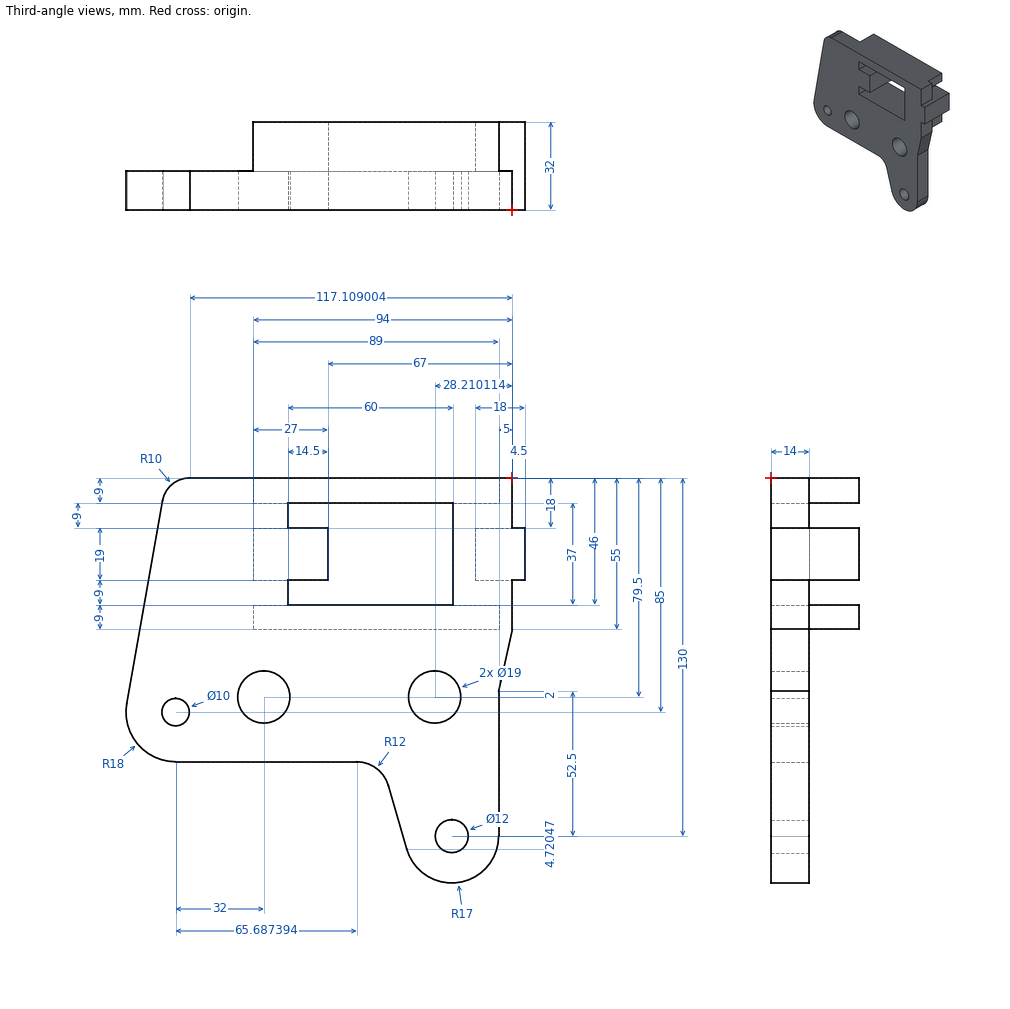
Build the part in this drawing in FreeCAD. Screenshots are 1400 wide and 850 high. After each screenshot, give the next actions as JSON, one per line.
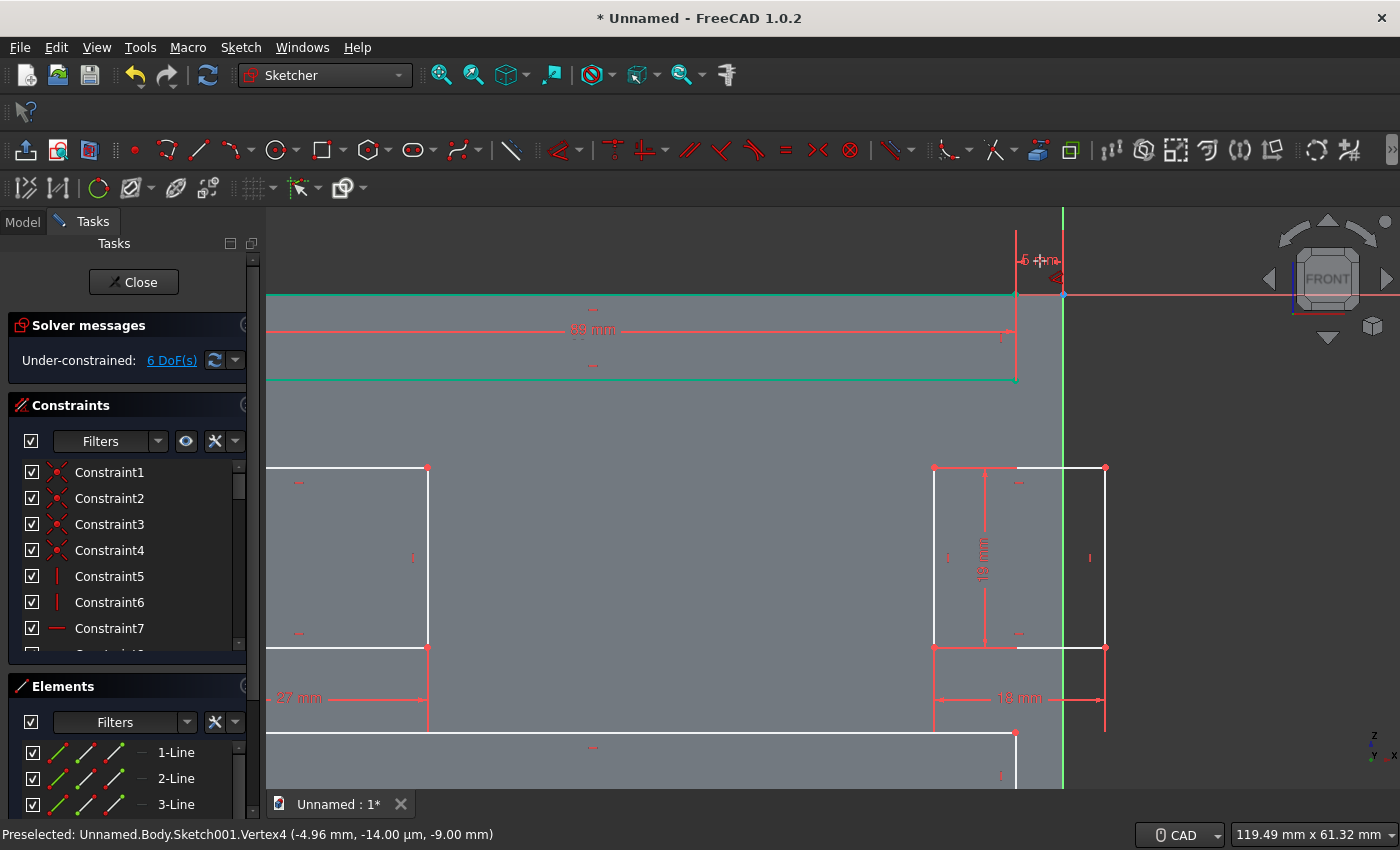
{"action": "scroll", "coordinate": [1021, 381], "scroll_direction": "down", "scroll_amount": 2}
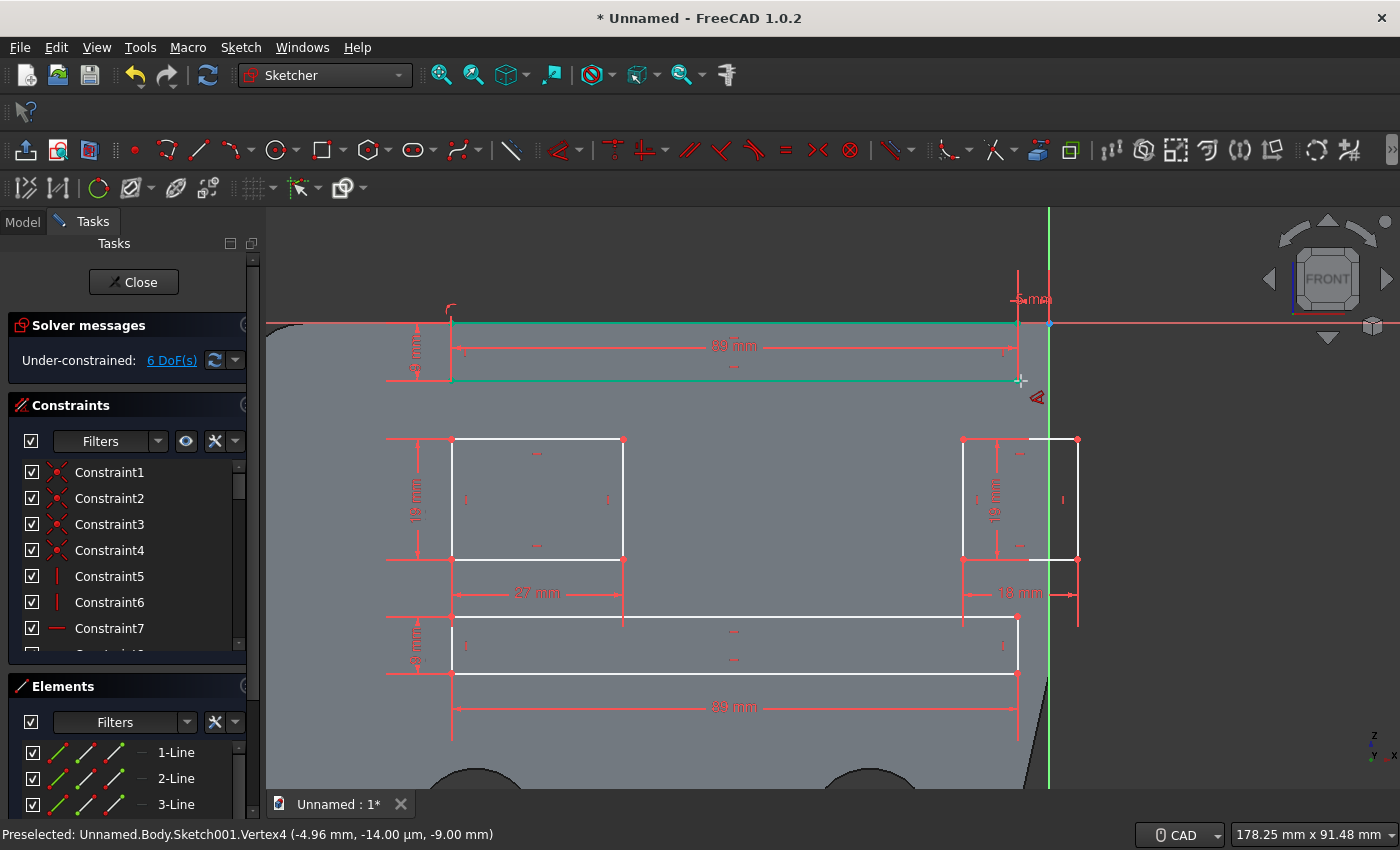
{"action": "scroll", "coordinate": [1018, 674], "scroll_direction": "up", "scroll_amount": 2}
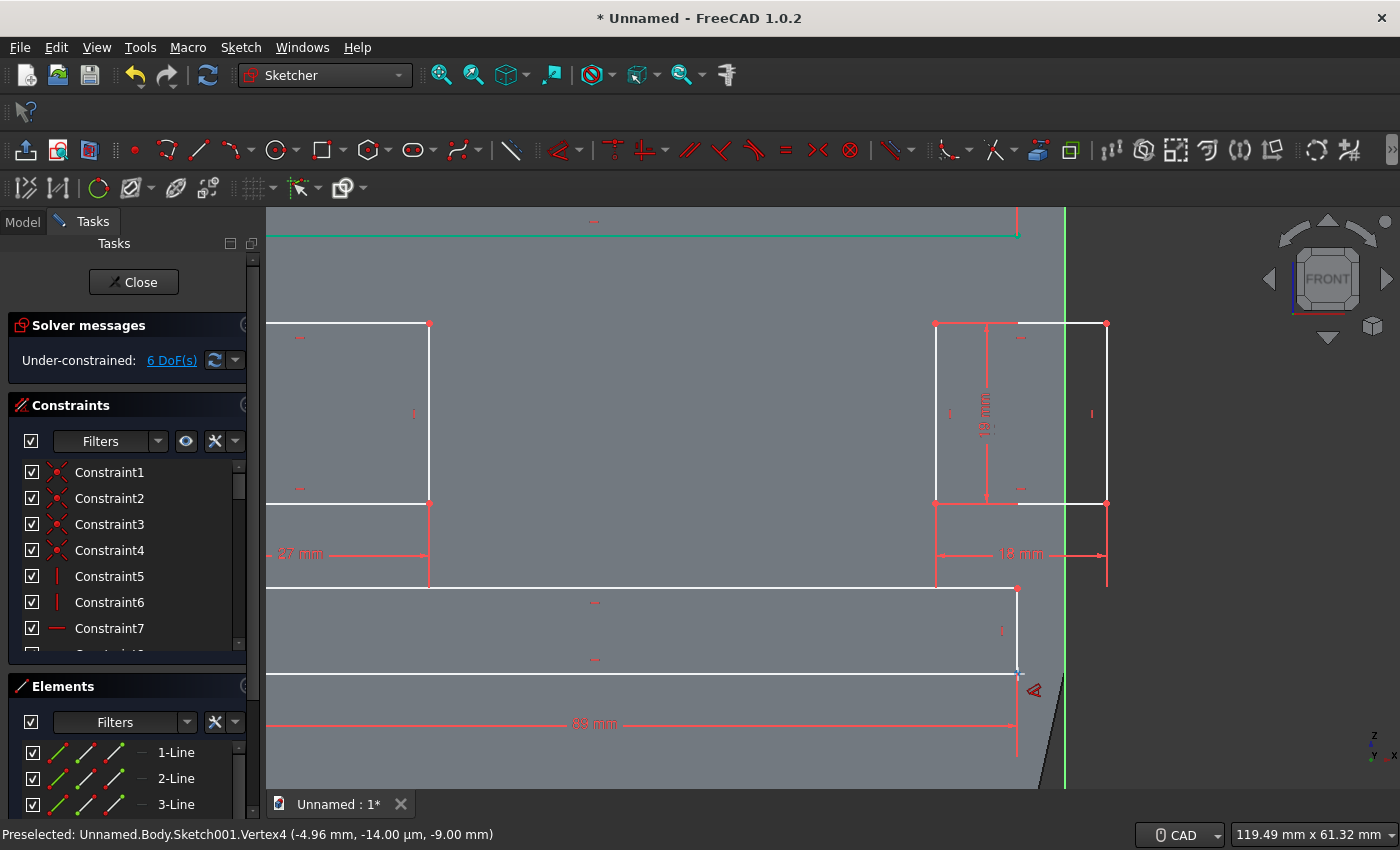
{"action": "left_click", "coordinate": [1017, 674]}
{"action": "left_click", "coordinate": [1041, 708]}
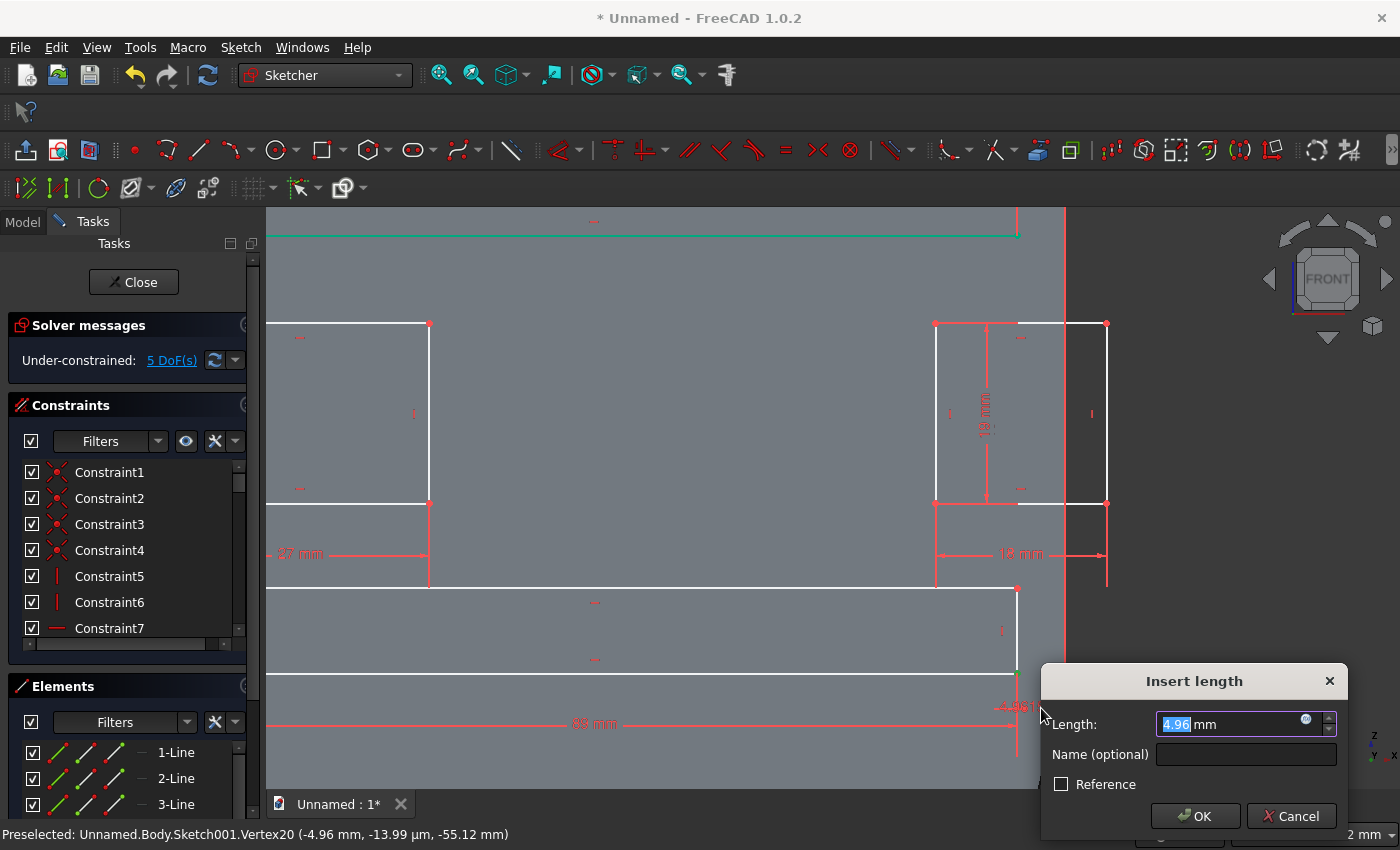
{"action": "type", "text": "5"}
{"action": "key", "text": "Return"}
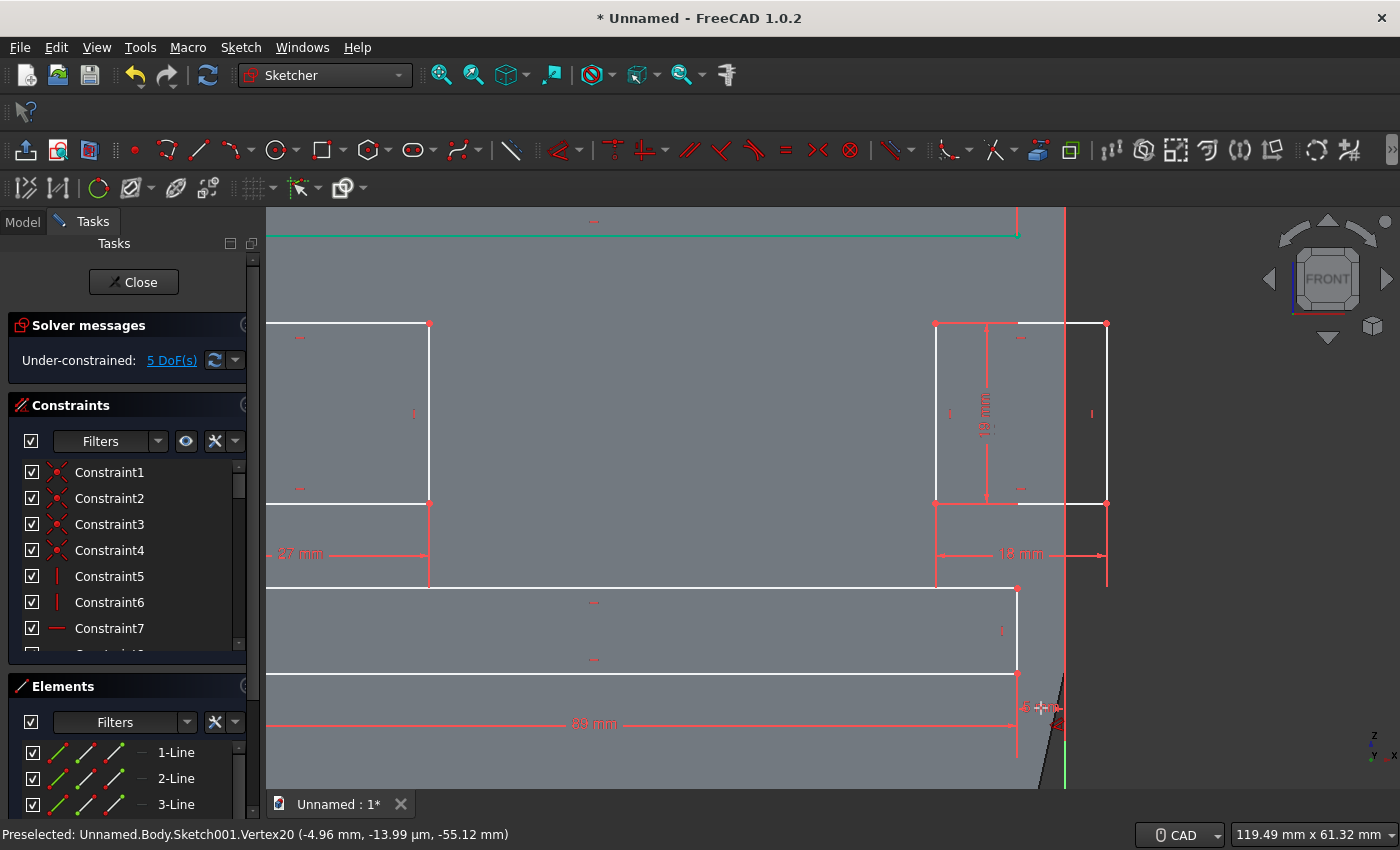
{"action": "scroll", "coordinate": [1018, 674], "scroll_direction": "down", "scroll_amount": 2}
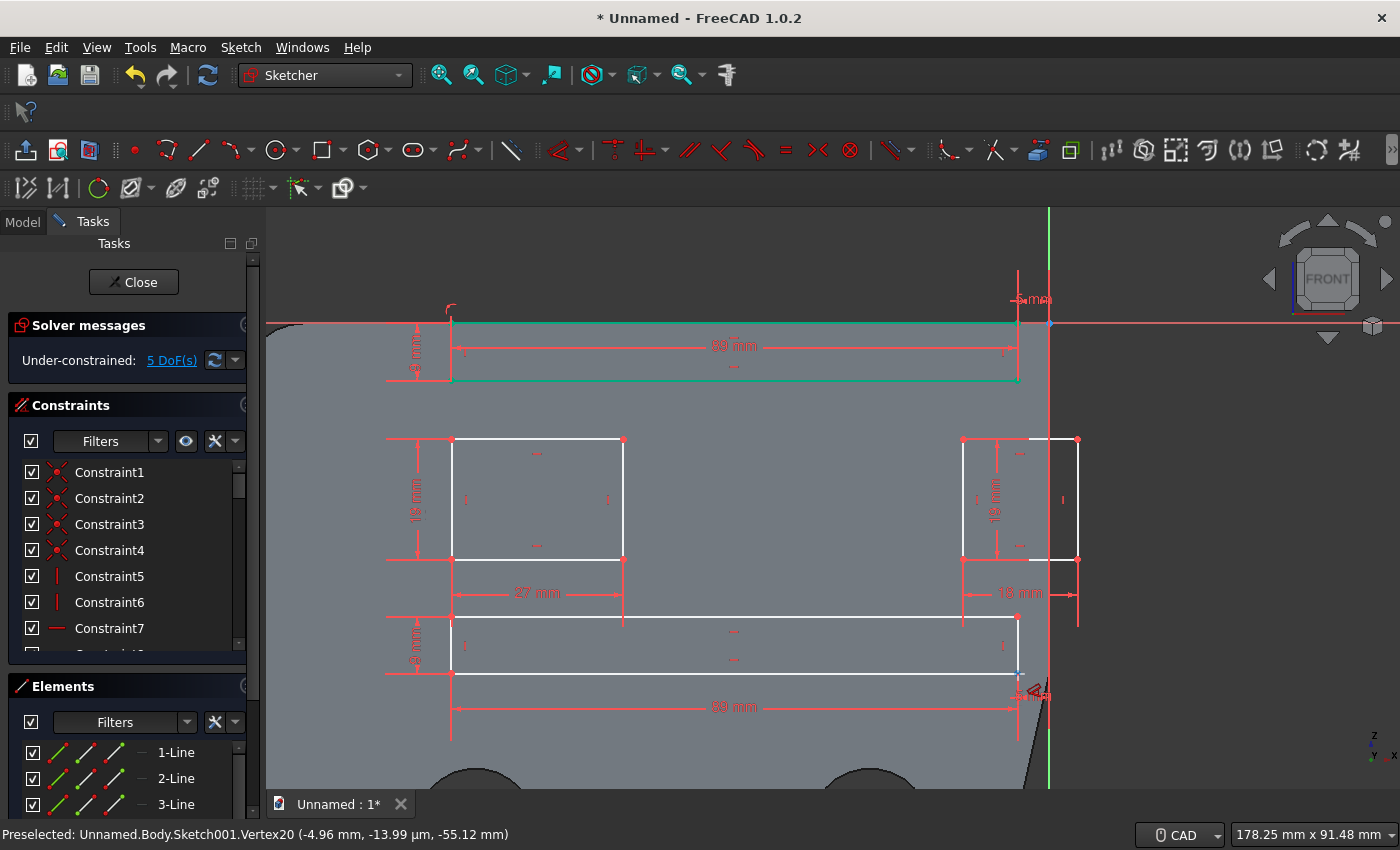
{"action": "left_click", "coordinate": [452, 439]}
{"action": "left_click", "coordinate": [751, 289]}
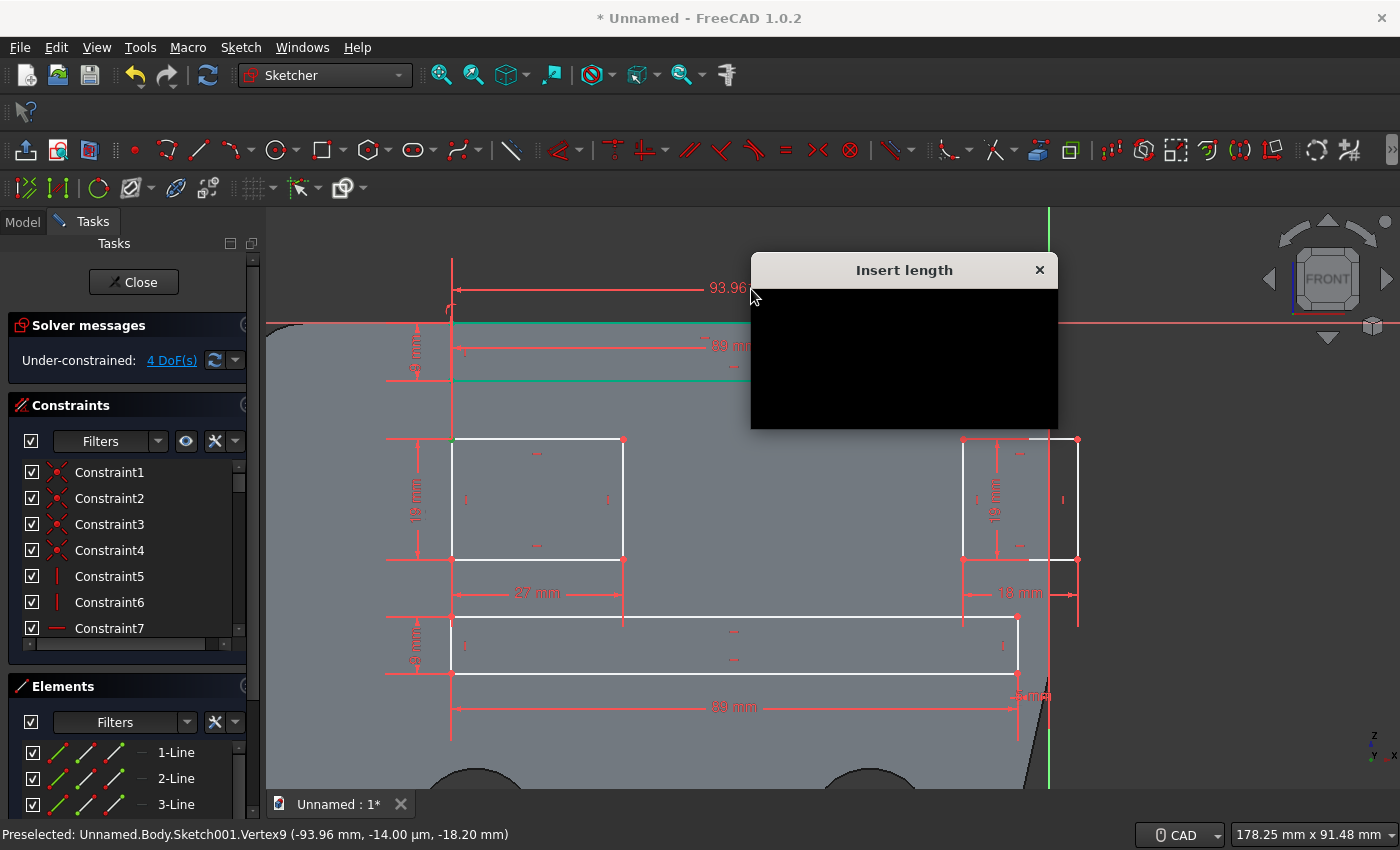
{"action": "type", "text": "94"}
{"action": "key", "text": "Return"}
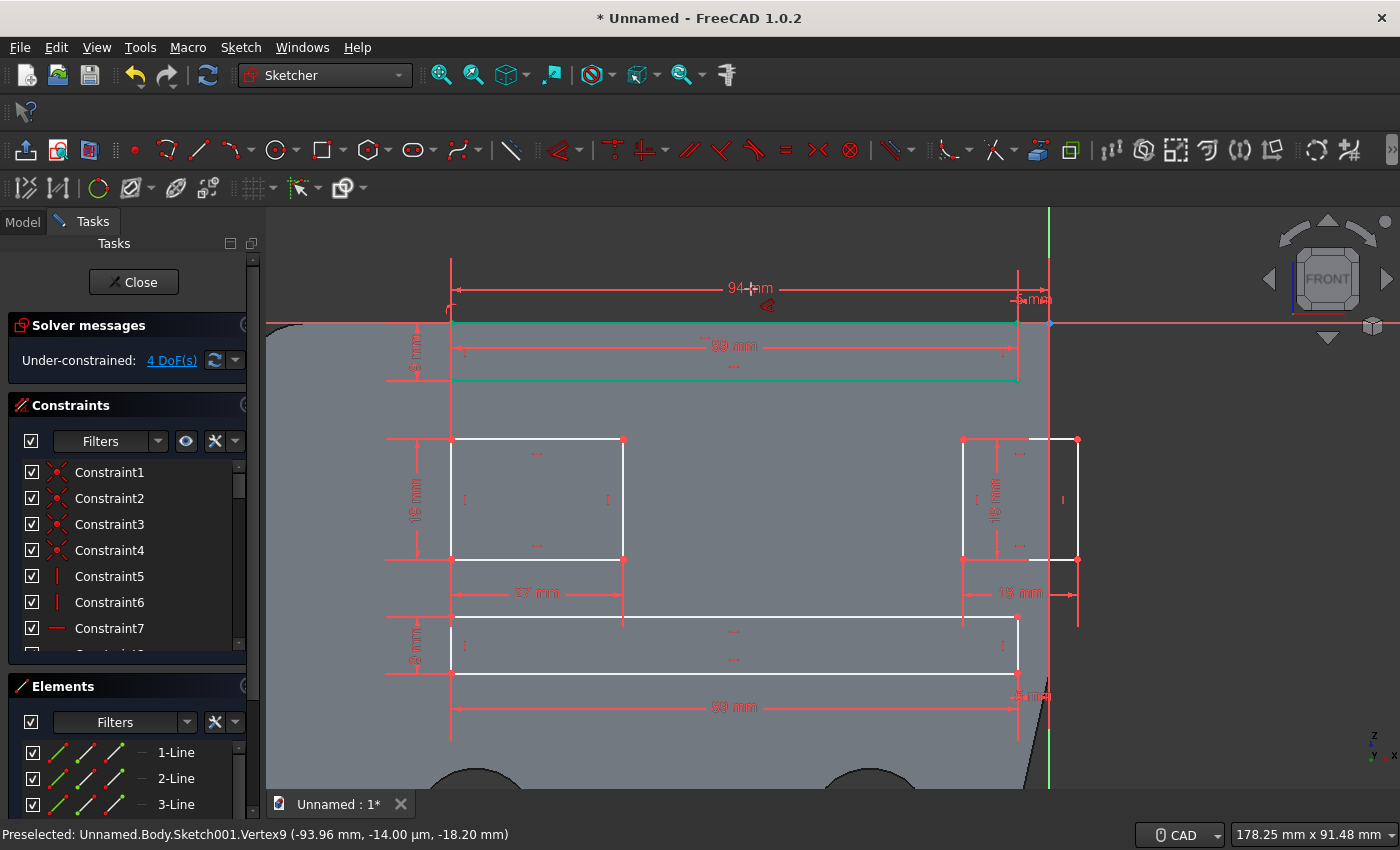
{"action": "left_click", "coordinate": [451, 439]}
{"action": "left_click", "coordinate": [417, 381]}